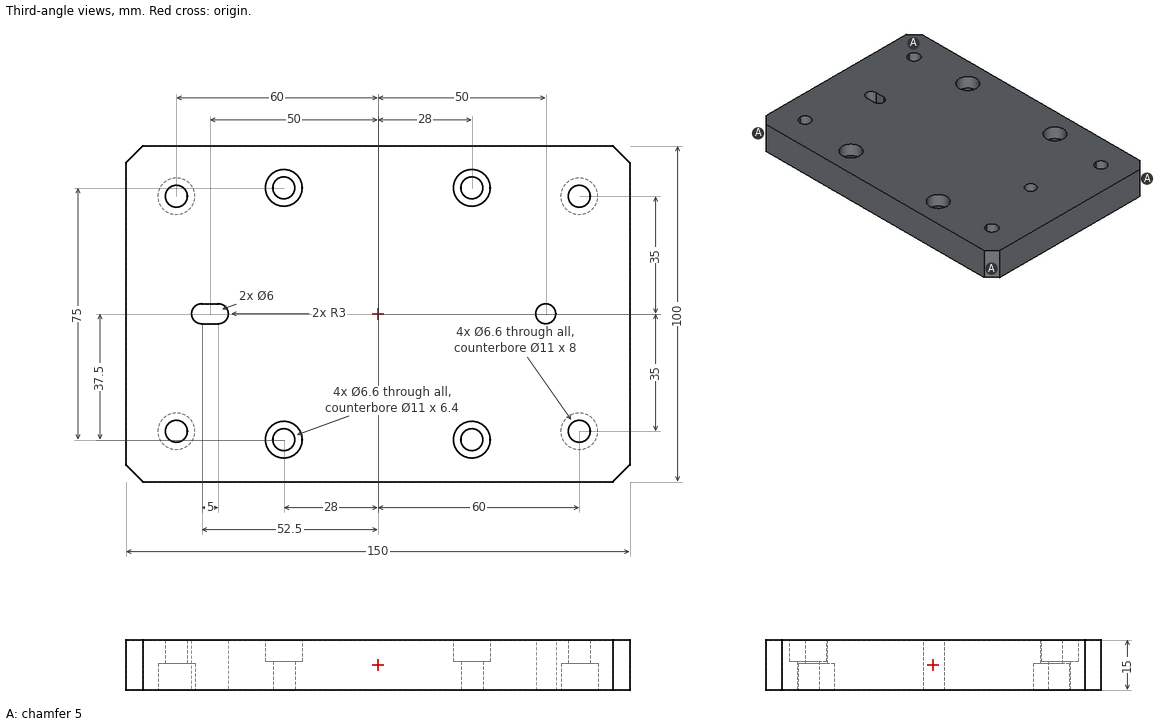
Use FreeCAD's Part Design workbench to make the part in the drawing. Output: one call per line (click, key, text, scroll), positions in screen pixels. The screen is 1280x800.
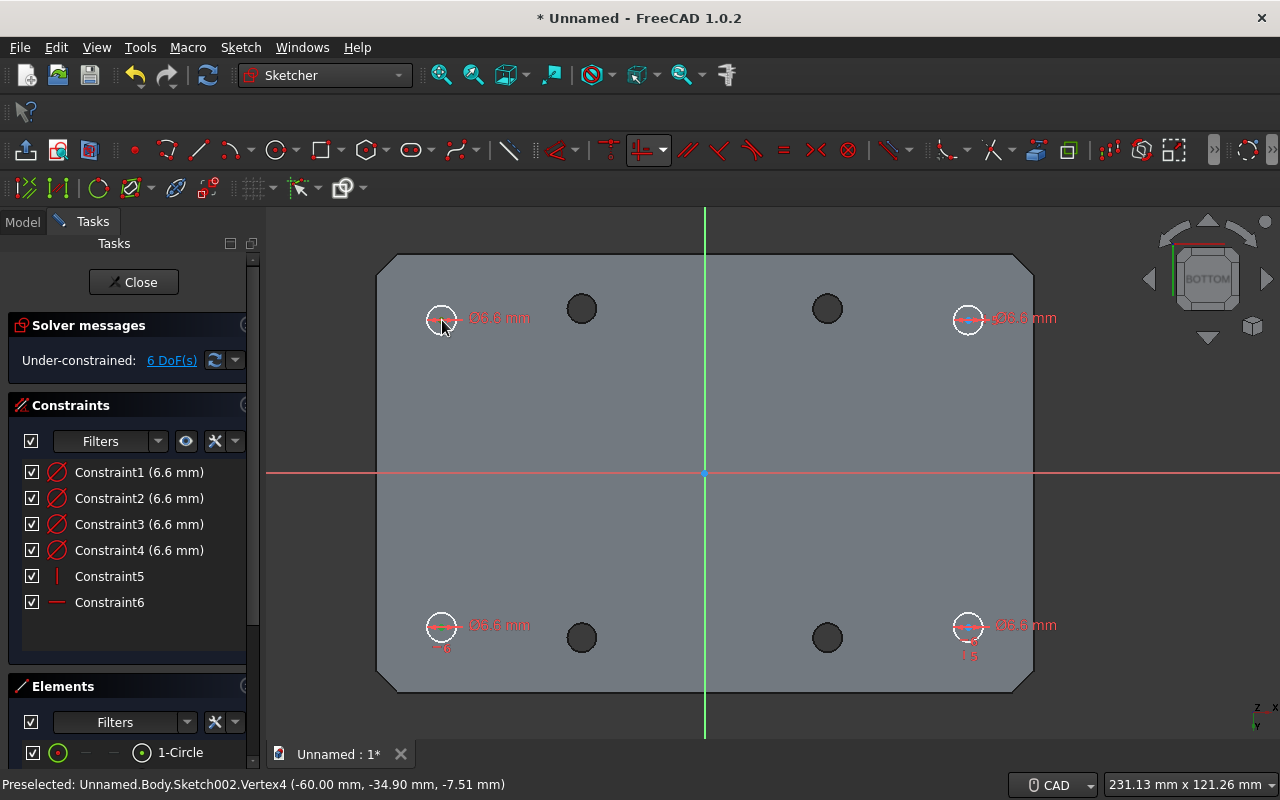
key(v)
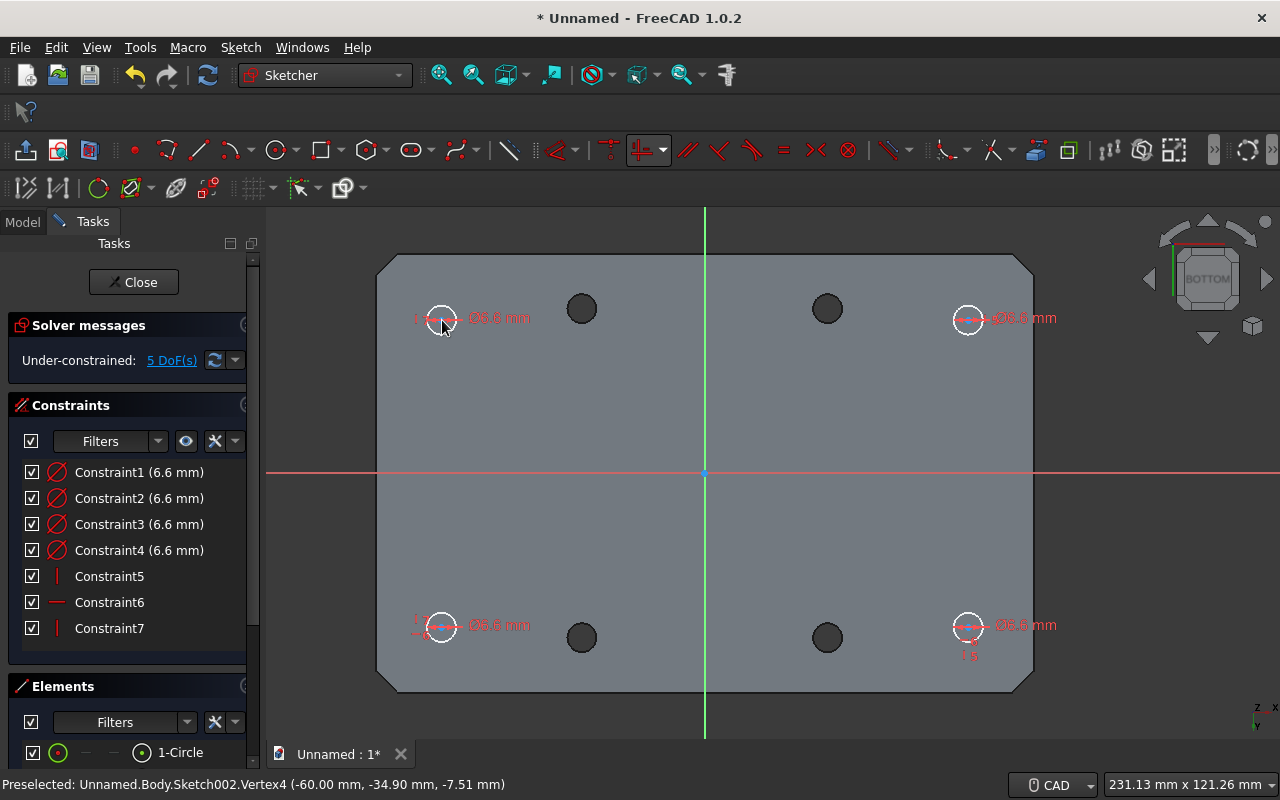
click(968, 320)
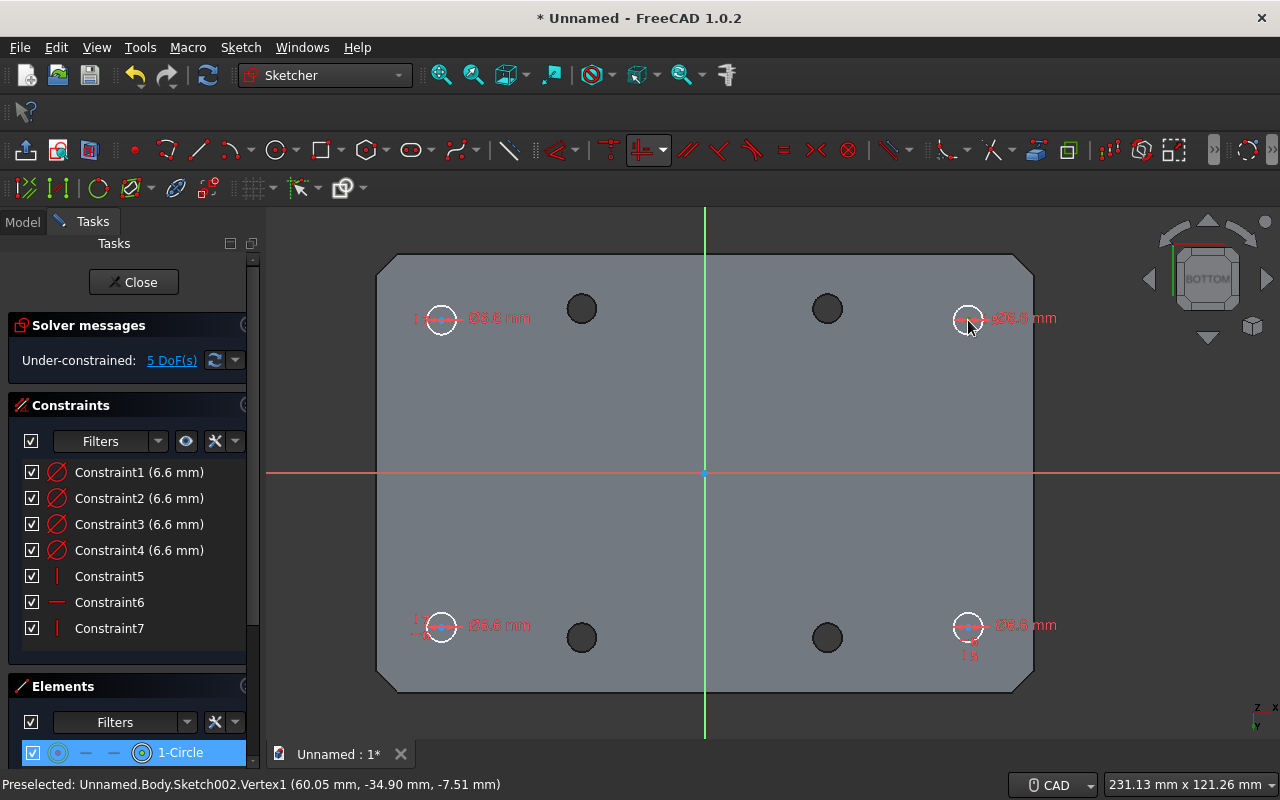
click(442, 320)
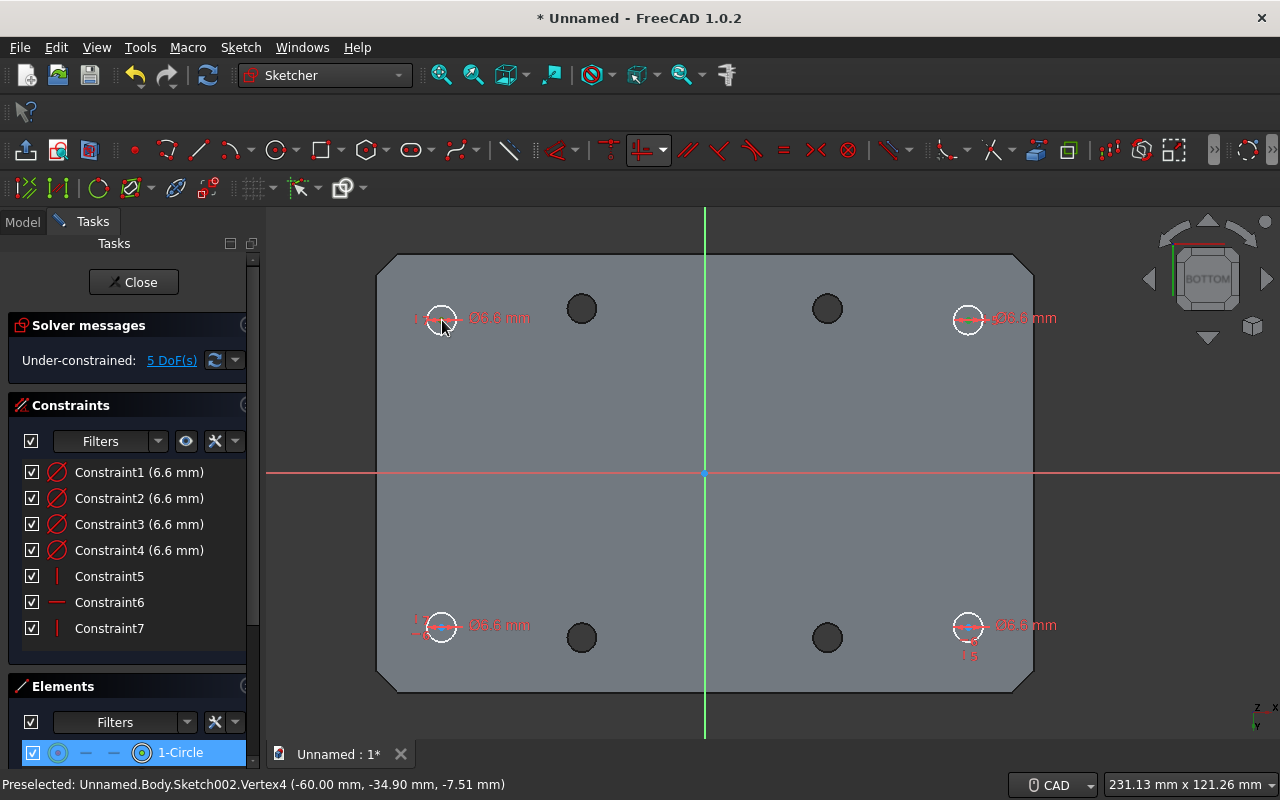
key(h)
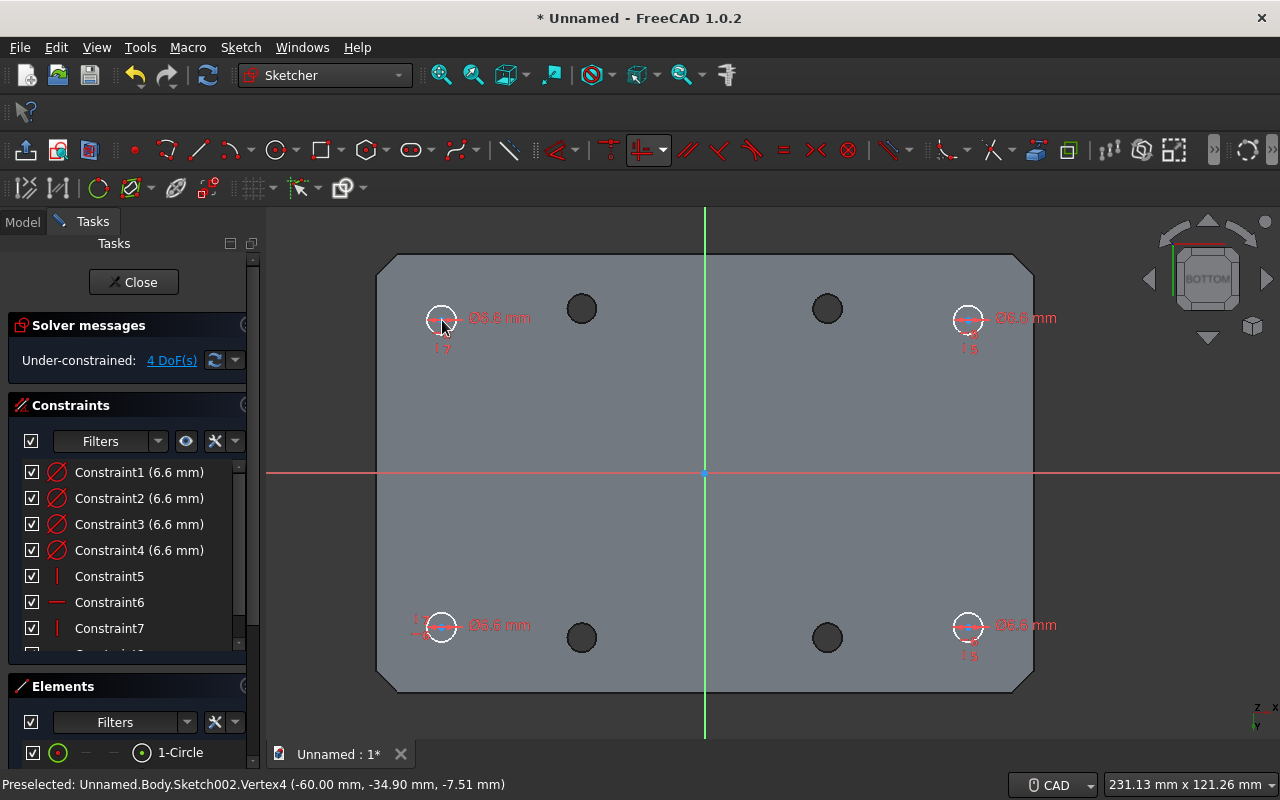
key(d)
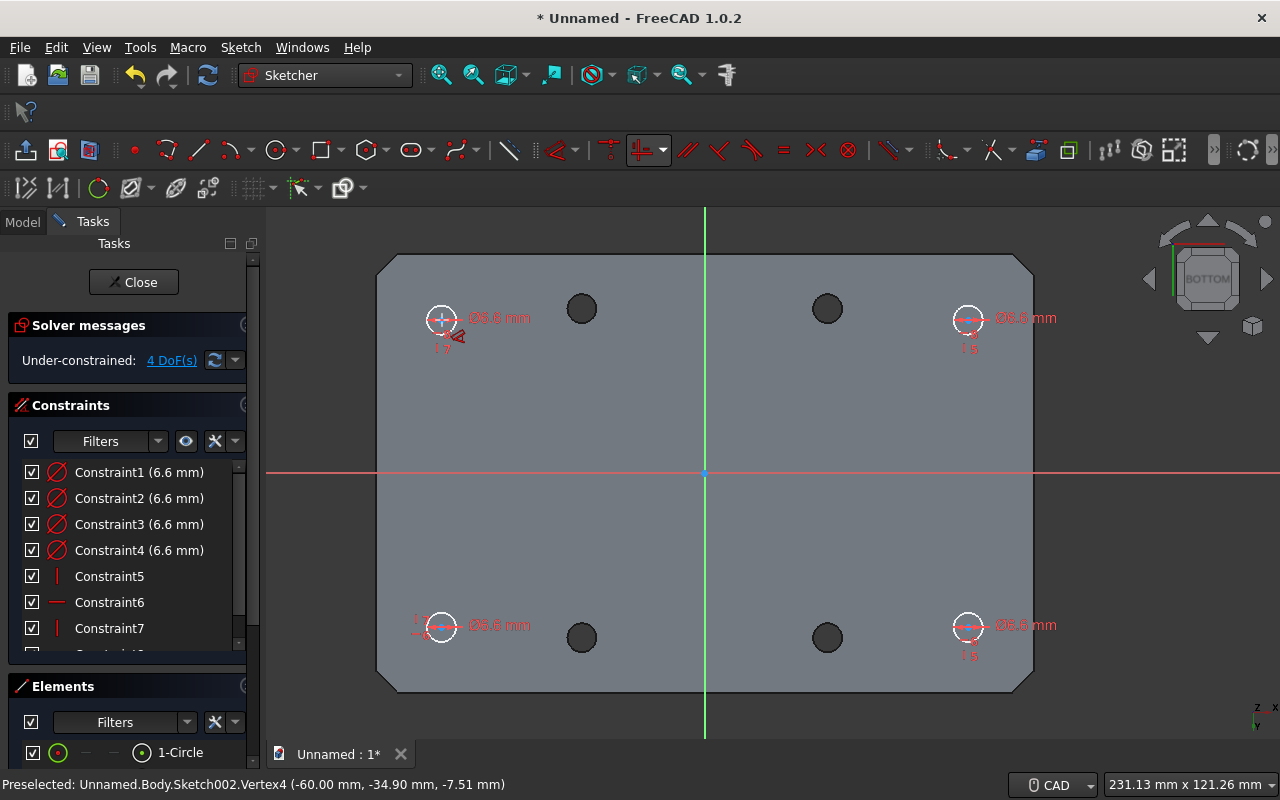
click(968, 320)
click(836, 286)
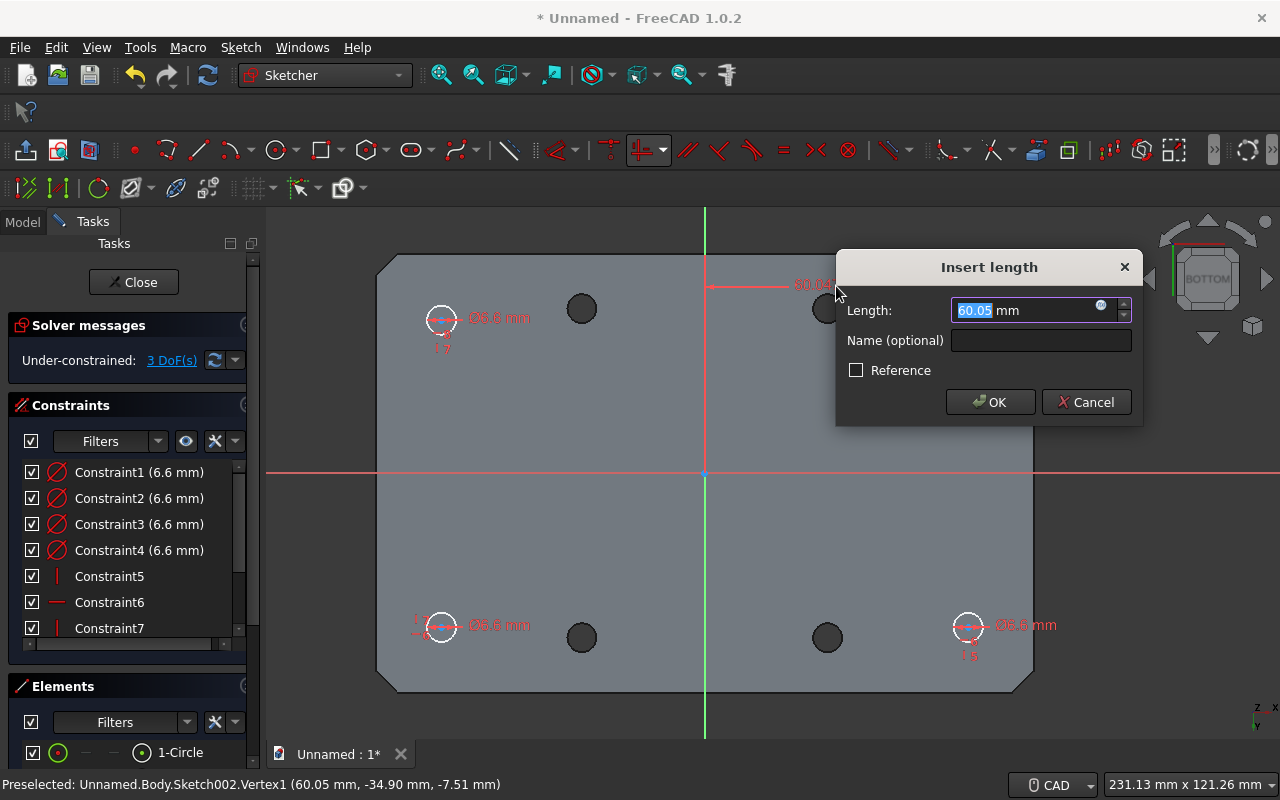
text(60)
key(Return)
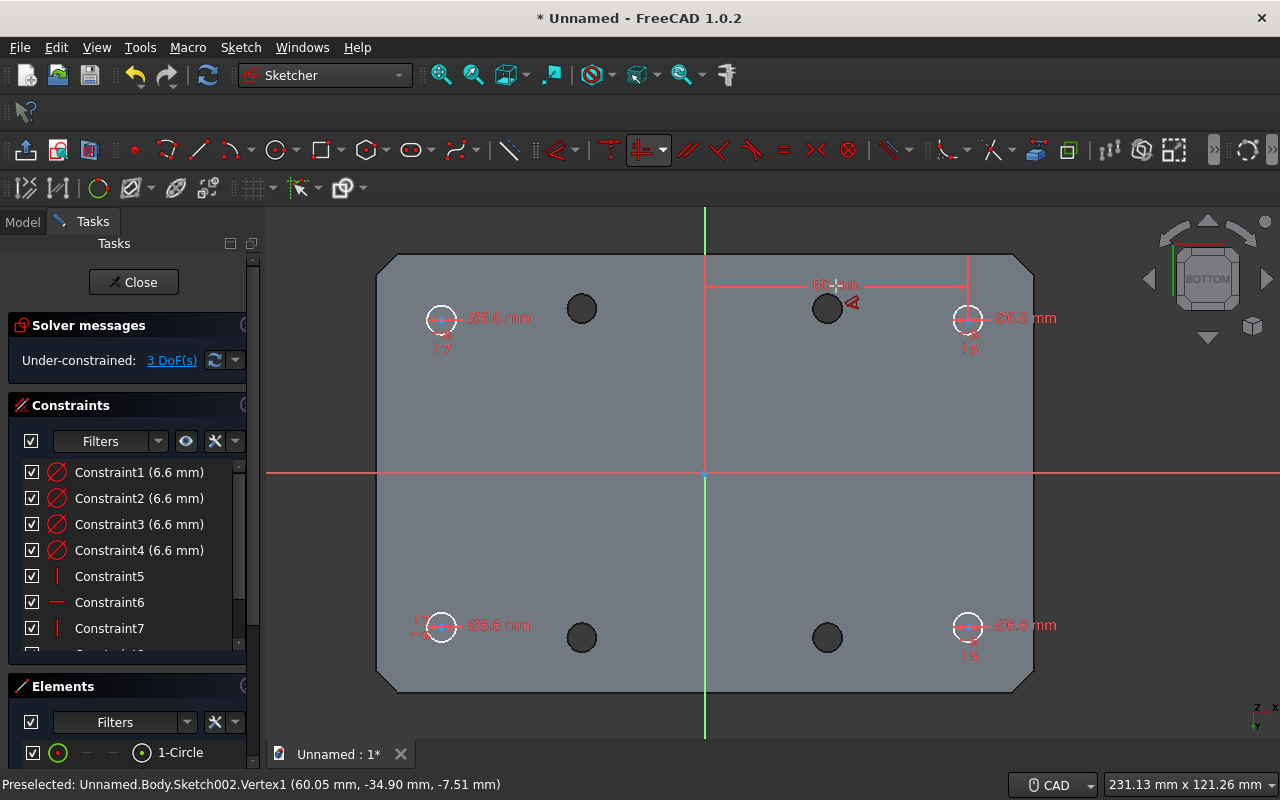
click(968, 320)
click(1002, 397)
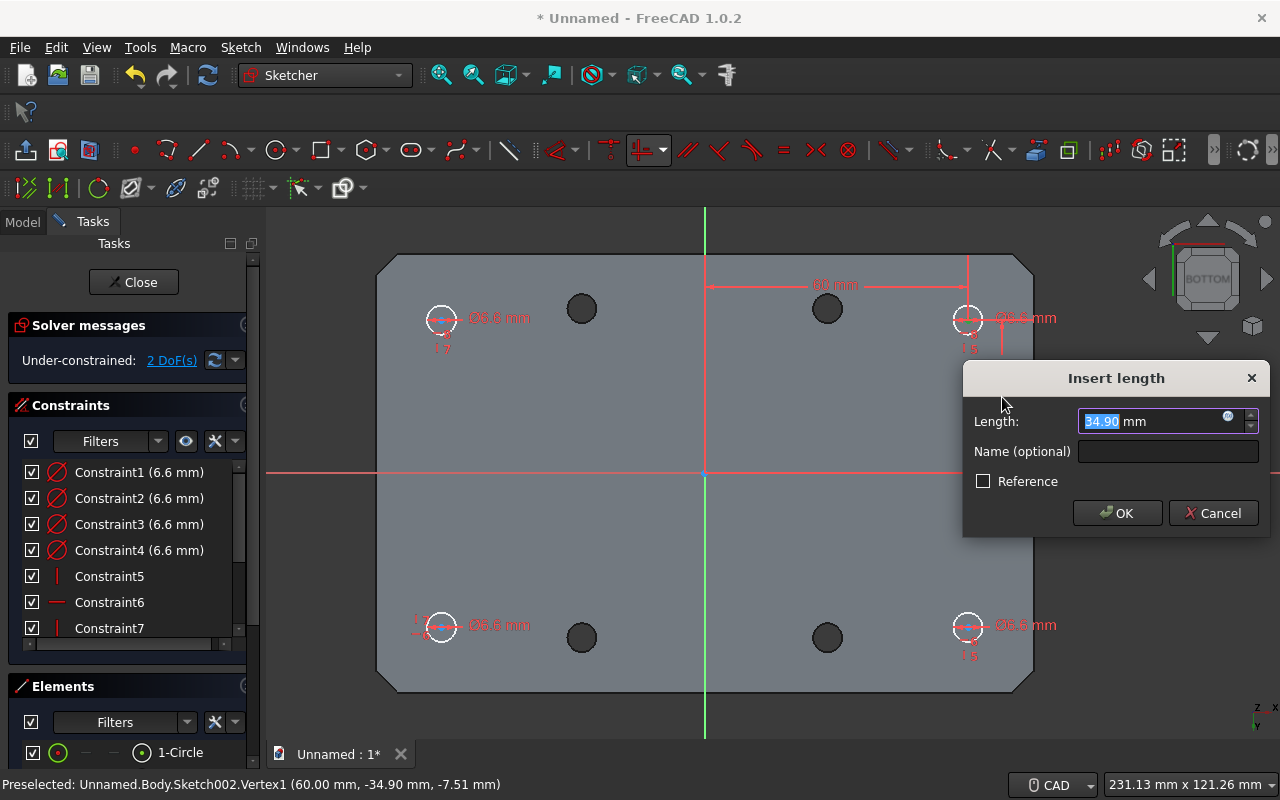
text(35)
key(Return)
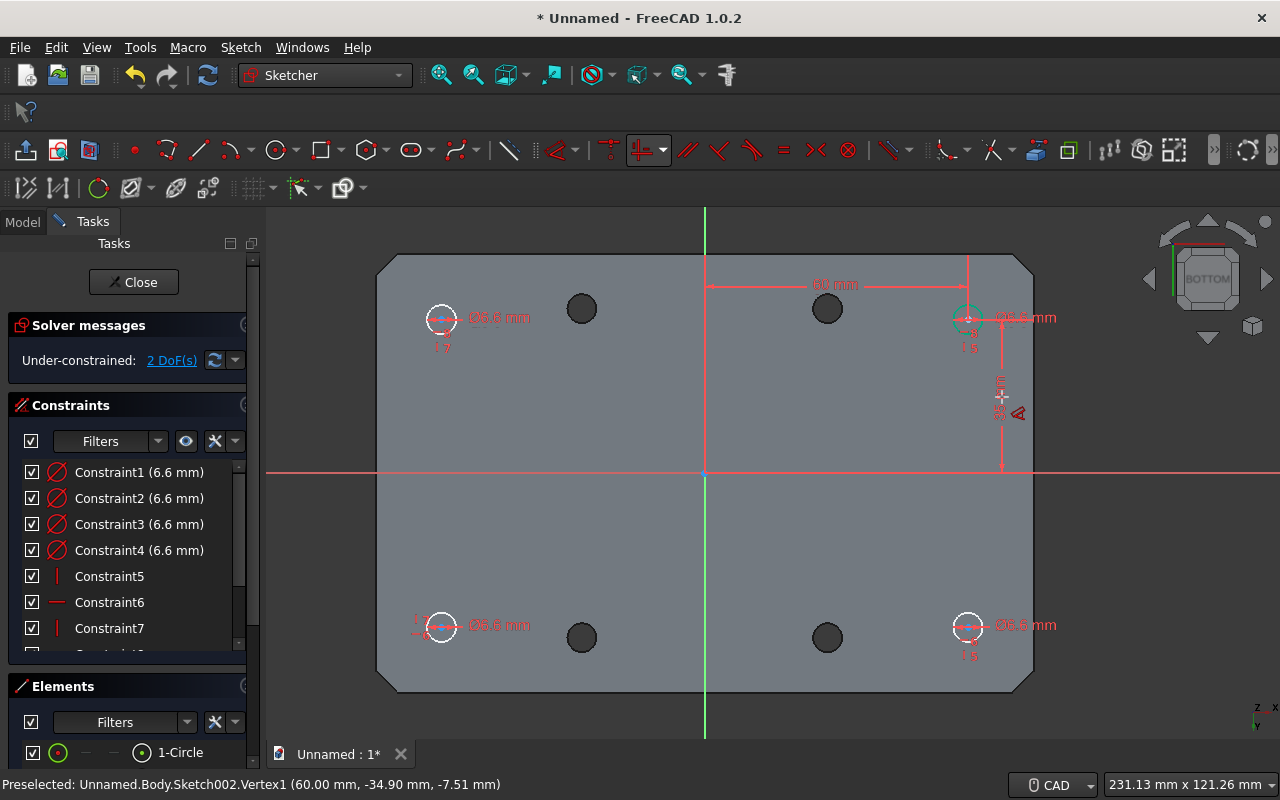
click(968, 627)
click(1002, 550)